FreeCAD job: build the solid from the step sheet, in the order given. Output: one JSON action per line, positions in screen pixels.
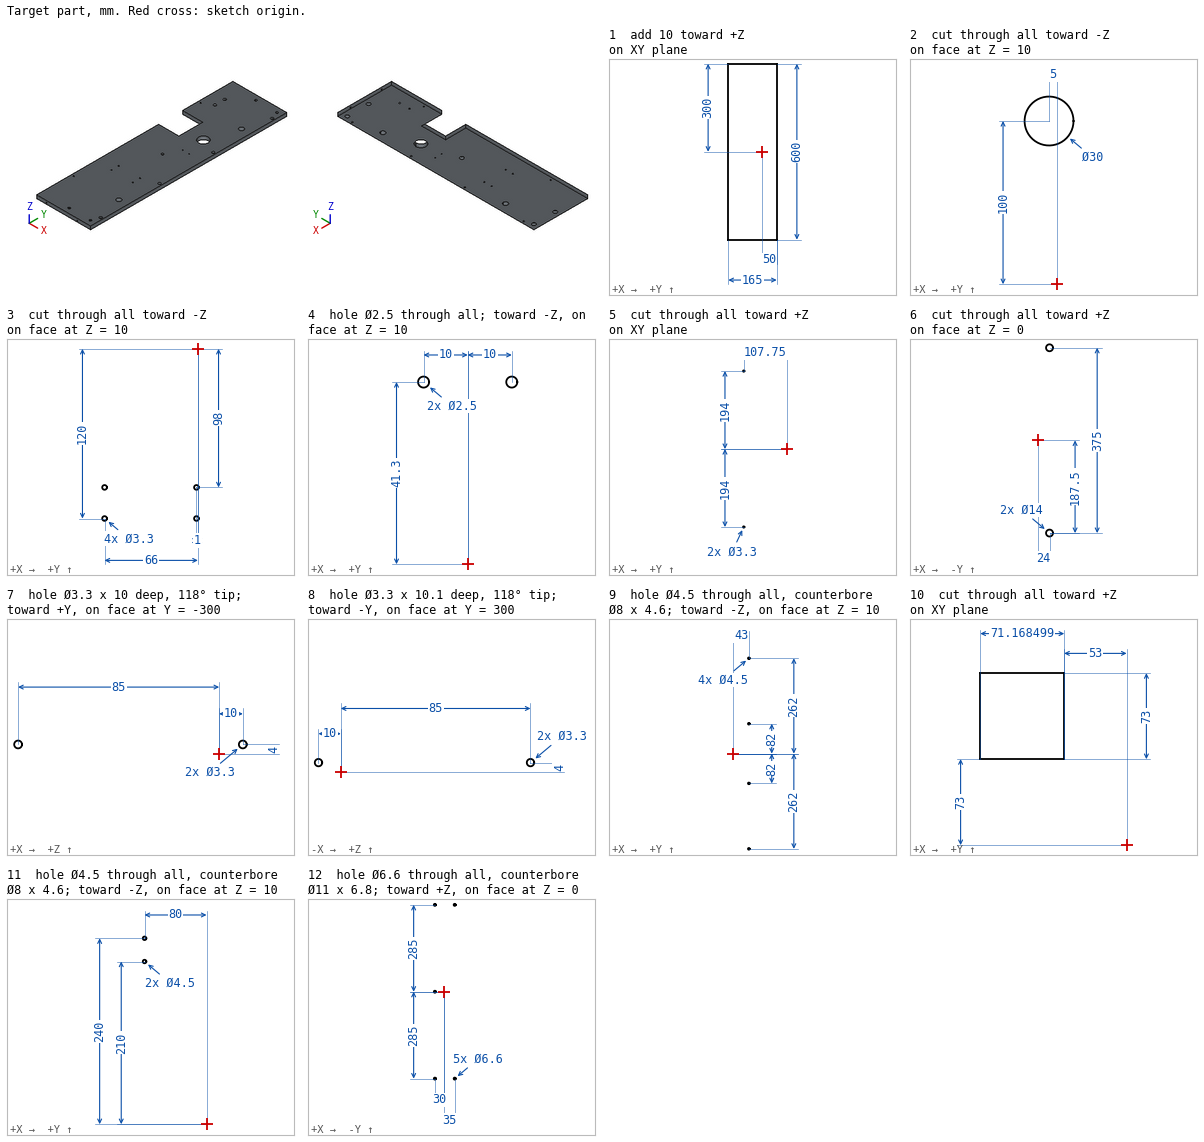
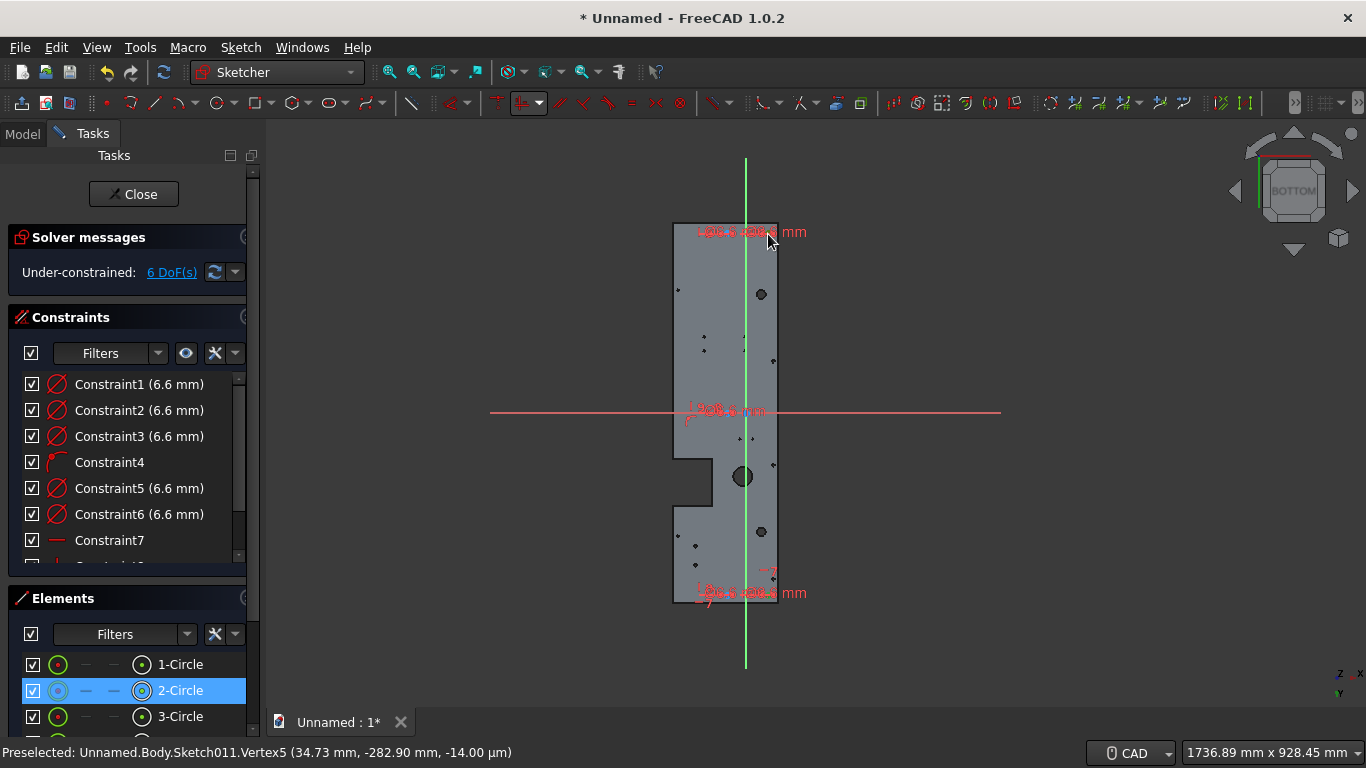
{"action": "key", "text": "v"}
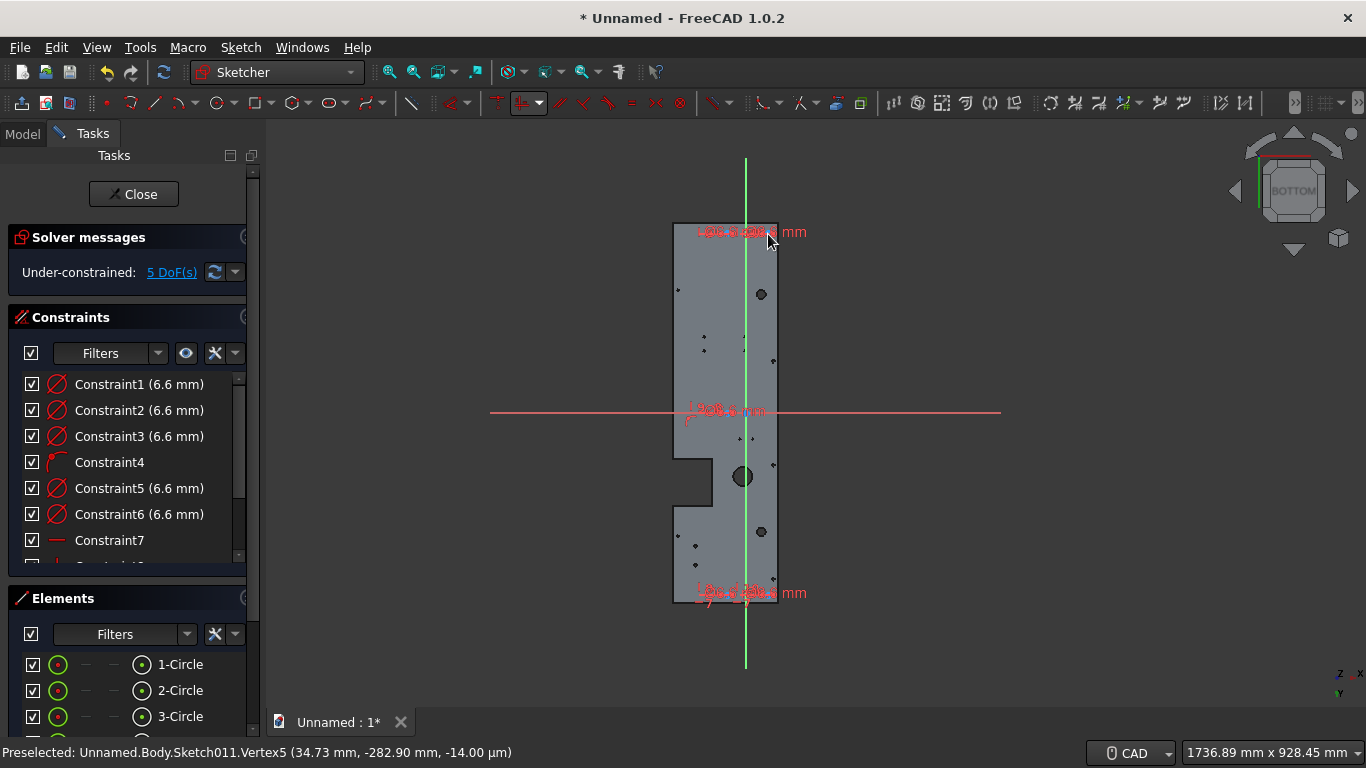
{"action": "left_click", "coordinate": [727, 234]}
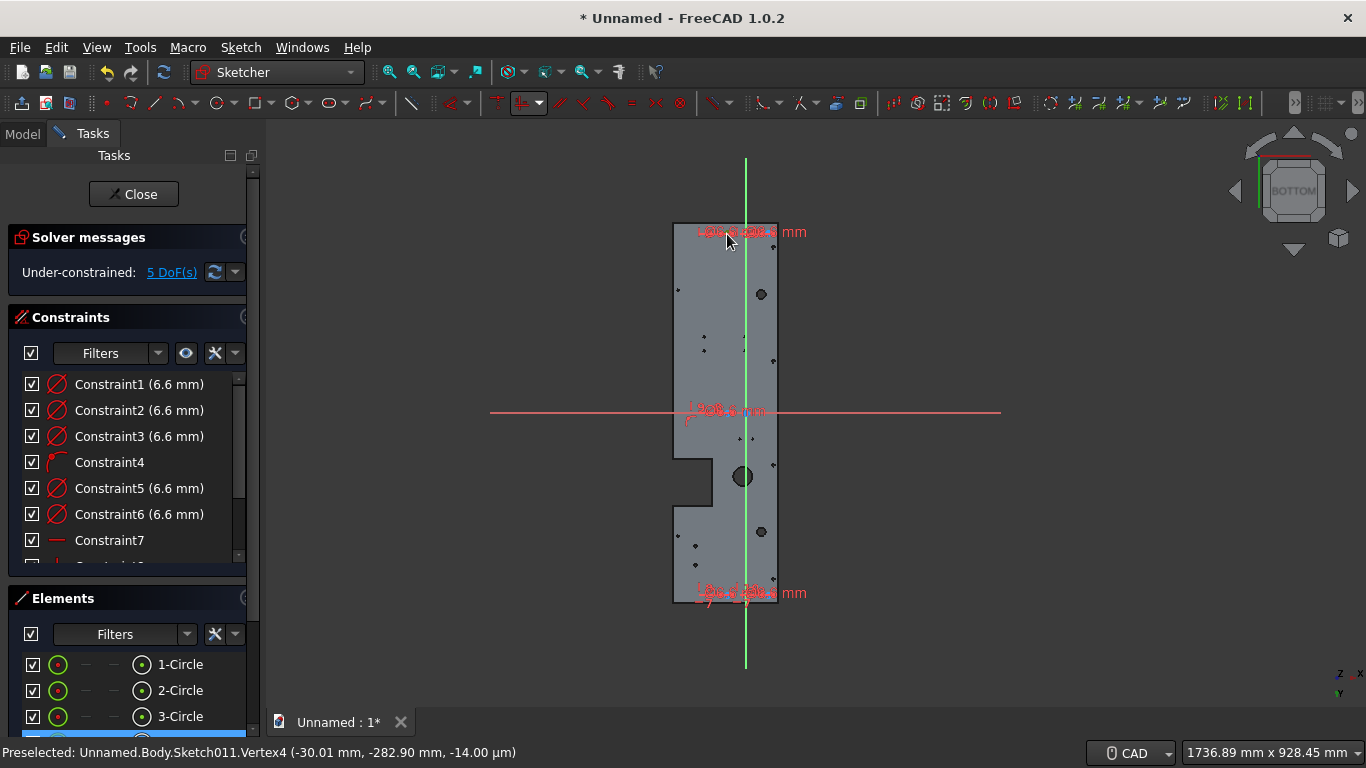
{"action": "left_click", "coordinate": [768, 234]}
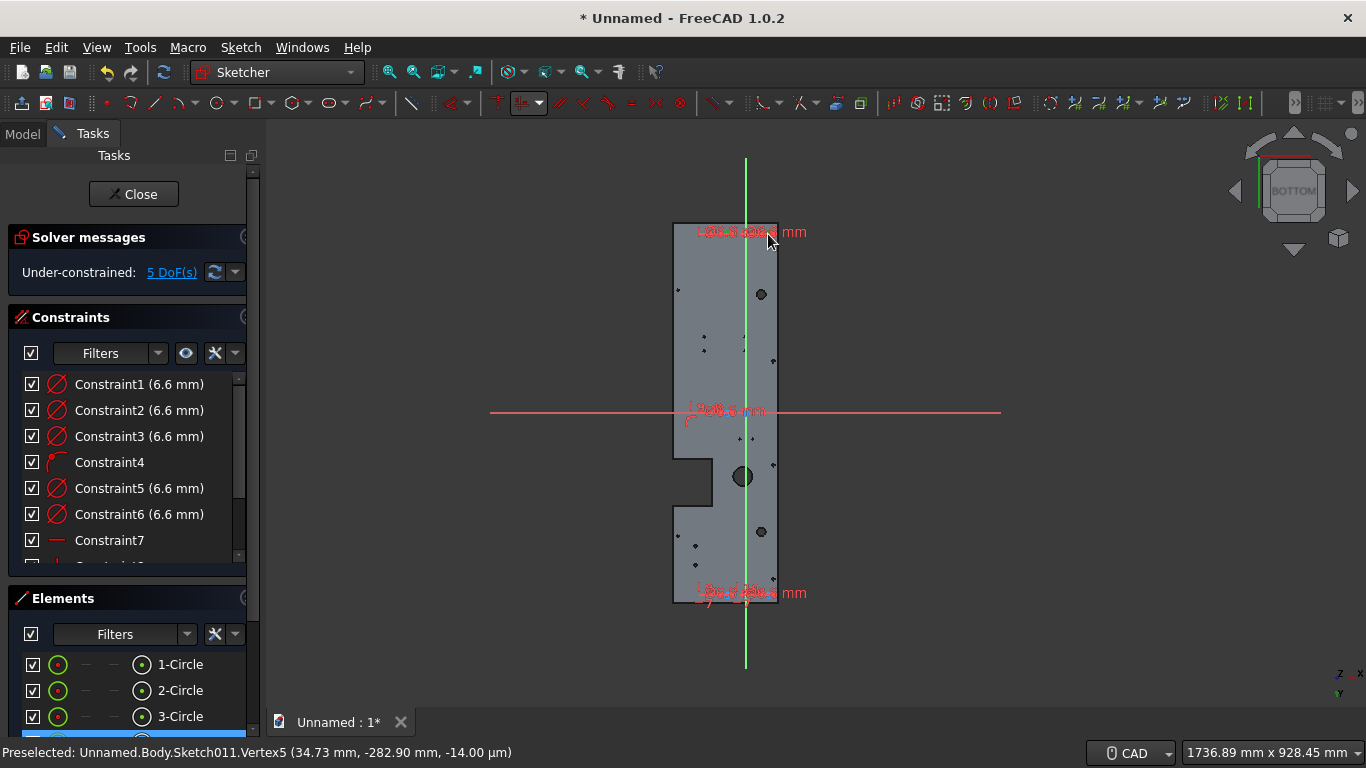
{"action": "left_click", "coordinate": [542, 104]}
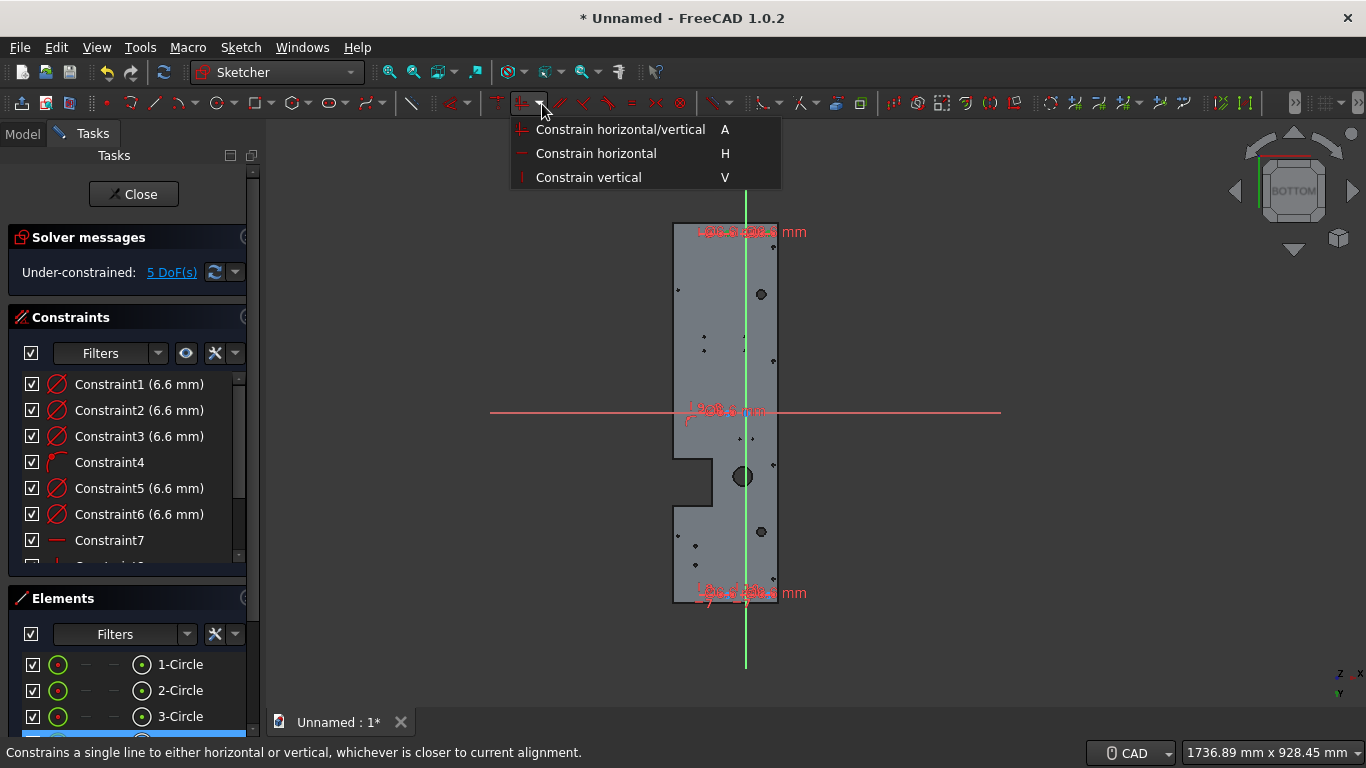
{"action": "left_click", "coordinate": [646, 153]}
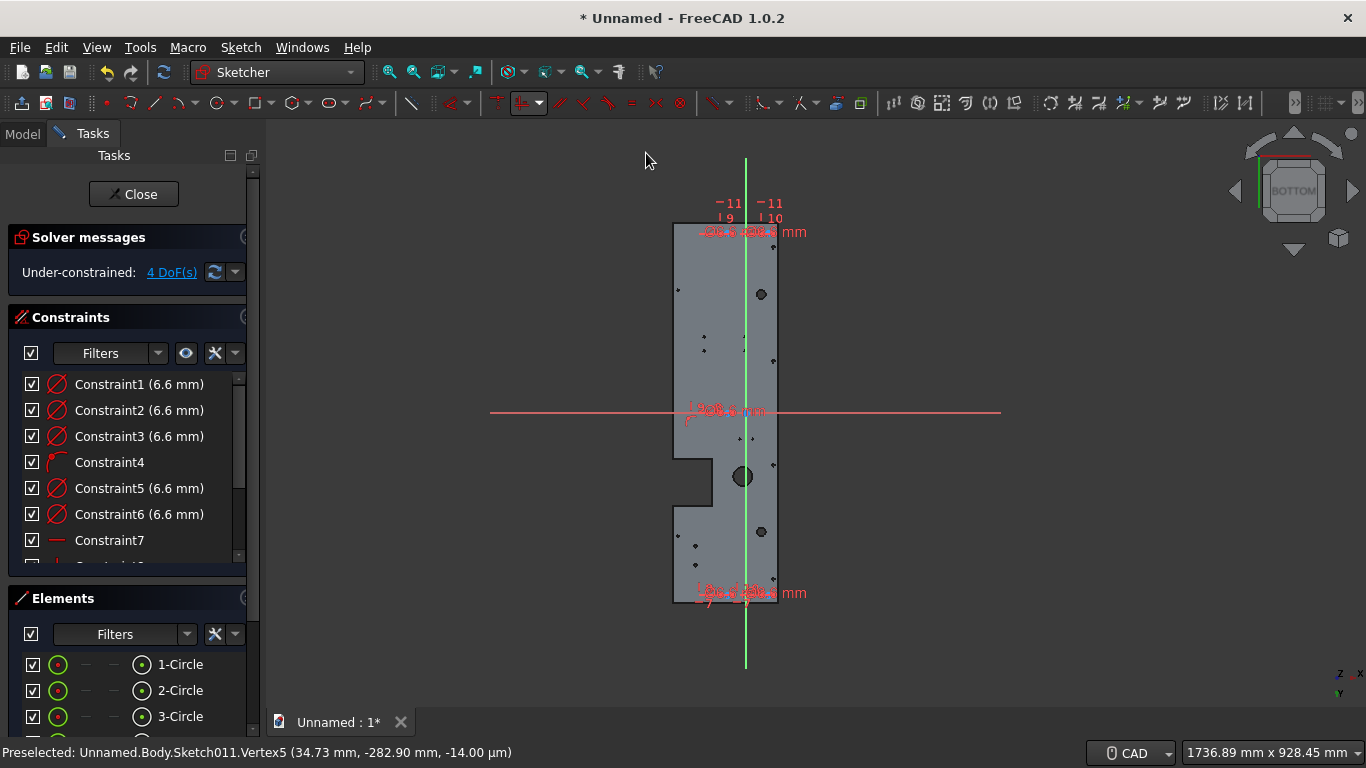
{"action": "left_click", "coordinate": [450, 104]}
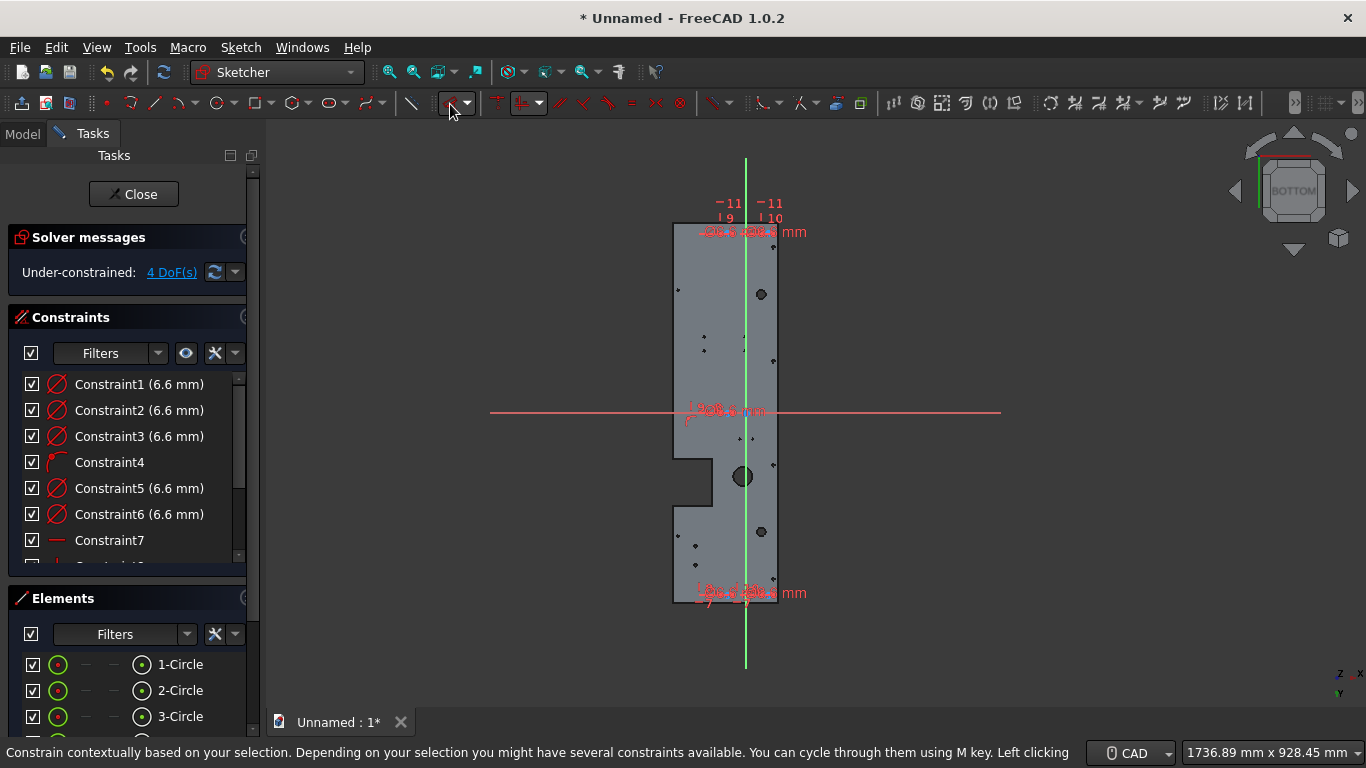
{"action": "scroll", "coordinate": [727, 595], "scroll_direction": "up", "scroll_amount": 4}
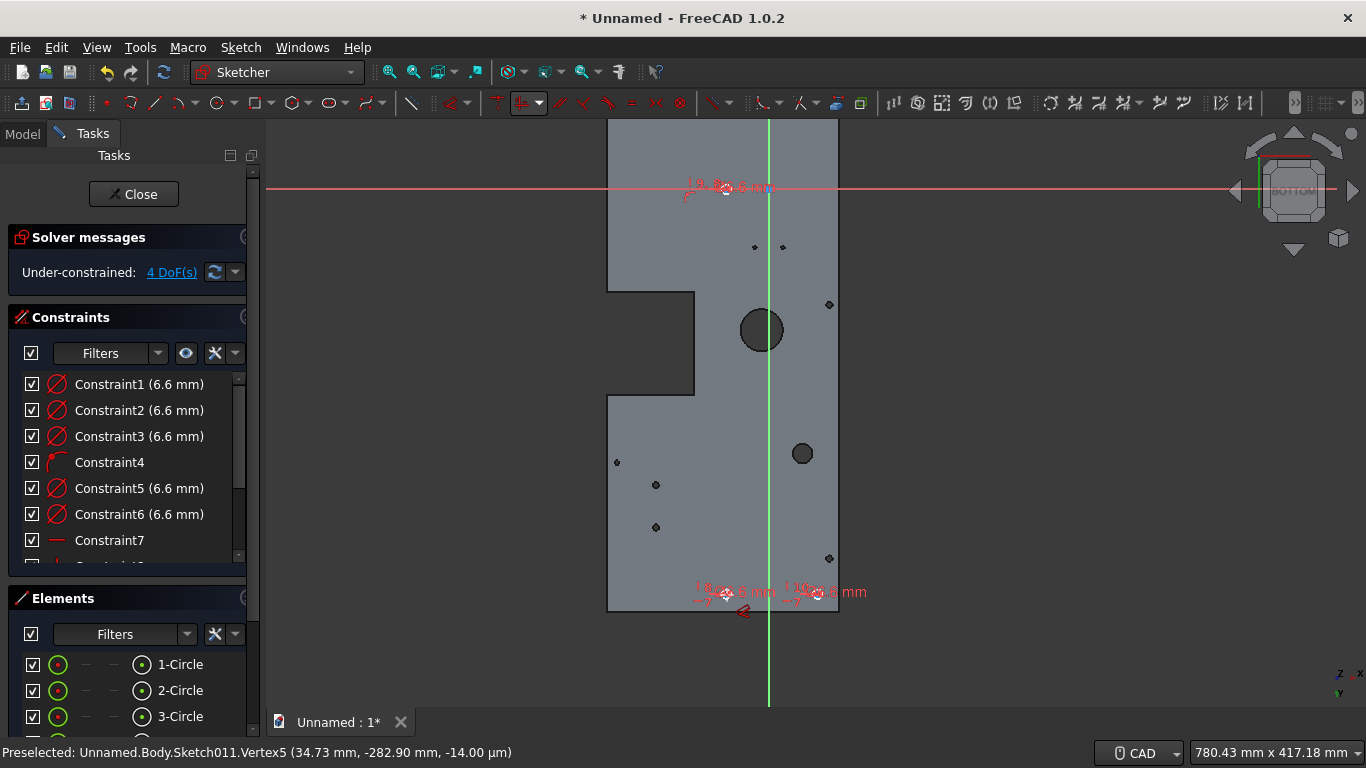
{"action": "left_click", "coordinate": [726, 594]}
{"action": "left_click", "coordinate": [748, 628]}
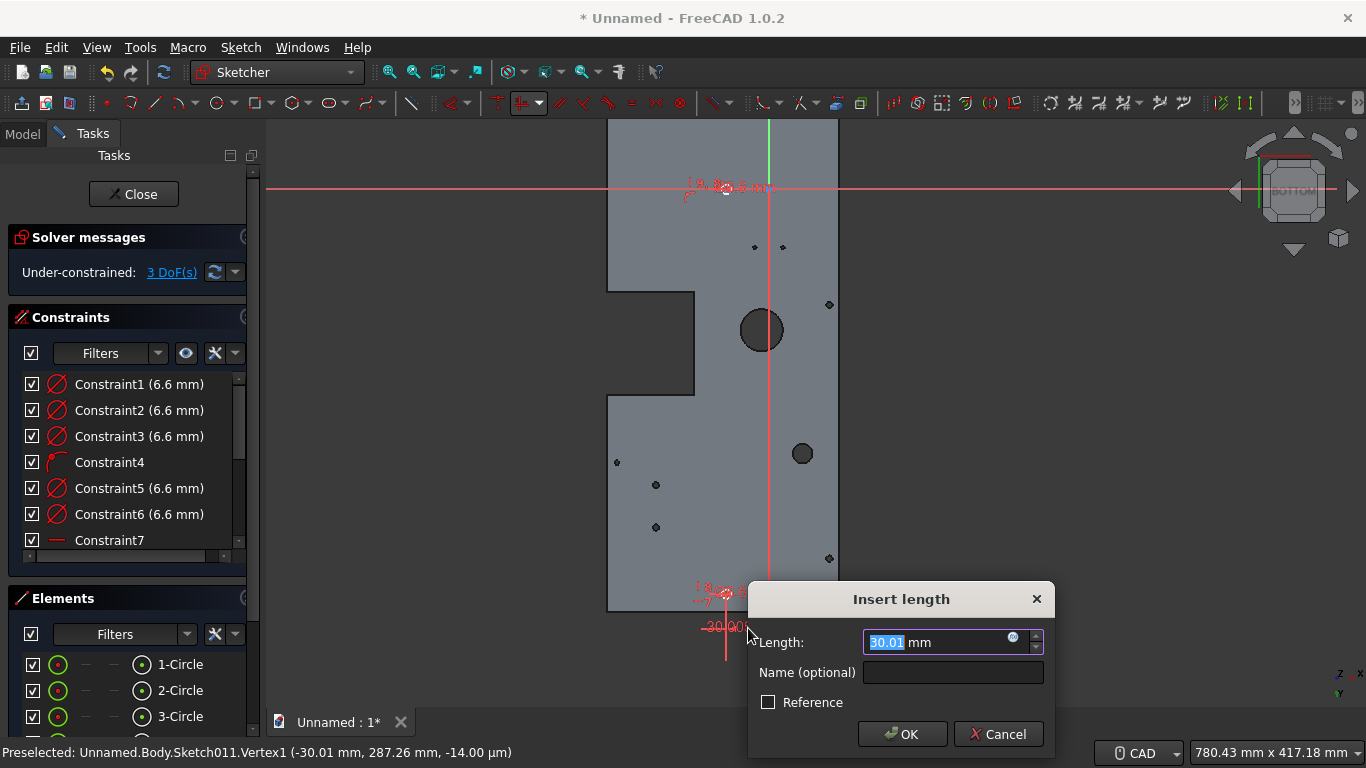
{"action": "type", "text": "30"}
{"action": "key", "text": "Return"}